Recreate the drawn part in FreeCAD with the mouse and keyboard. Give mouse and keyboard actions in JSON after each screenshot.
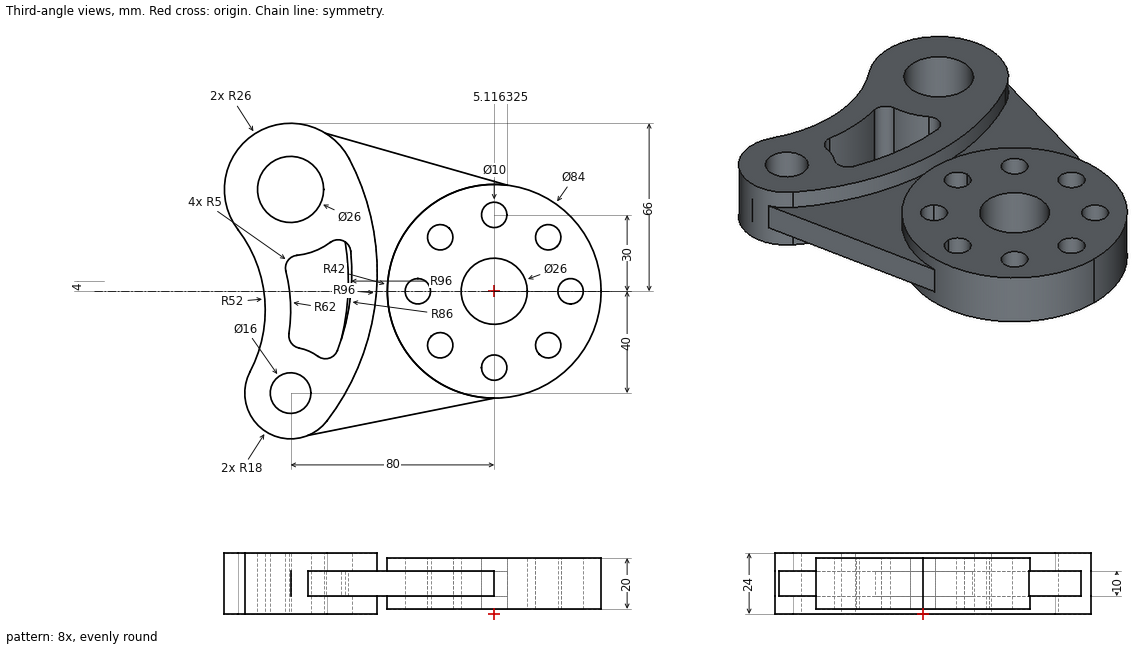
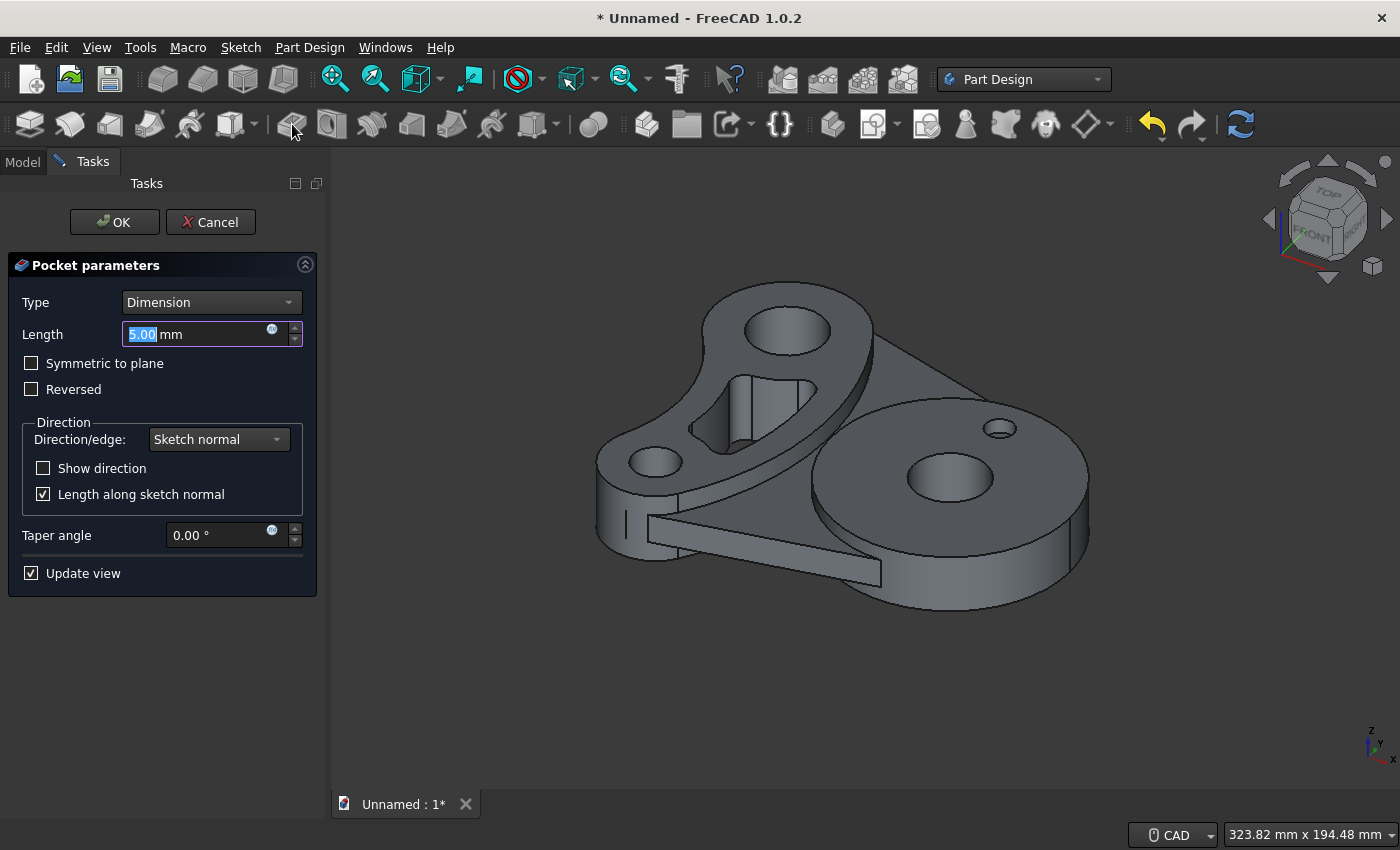
{"action": "left_click", "coordinate": [212, 302]}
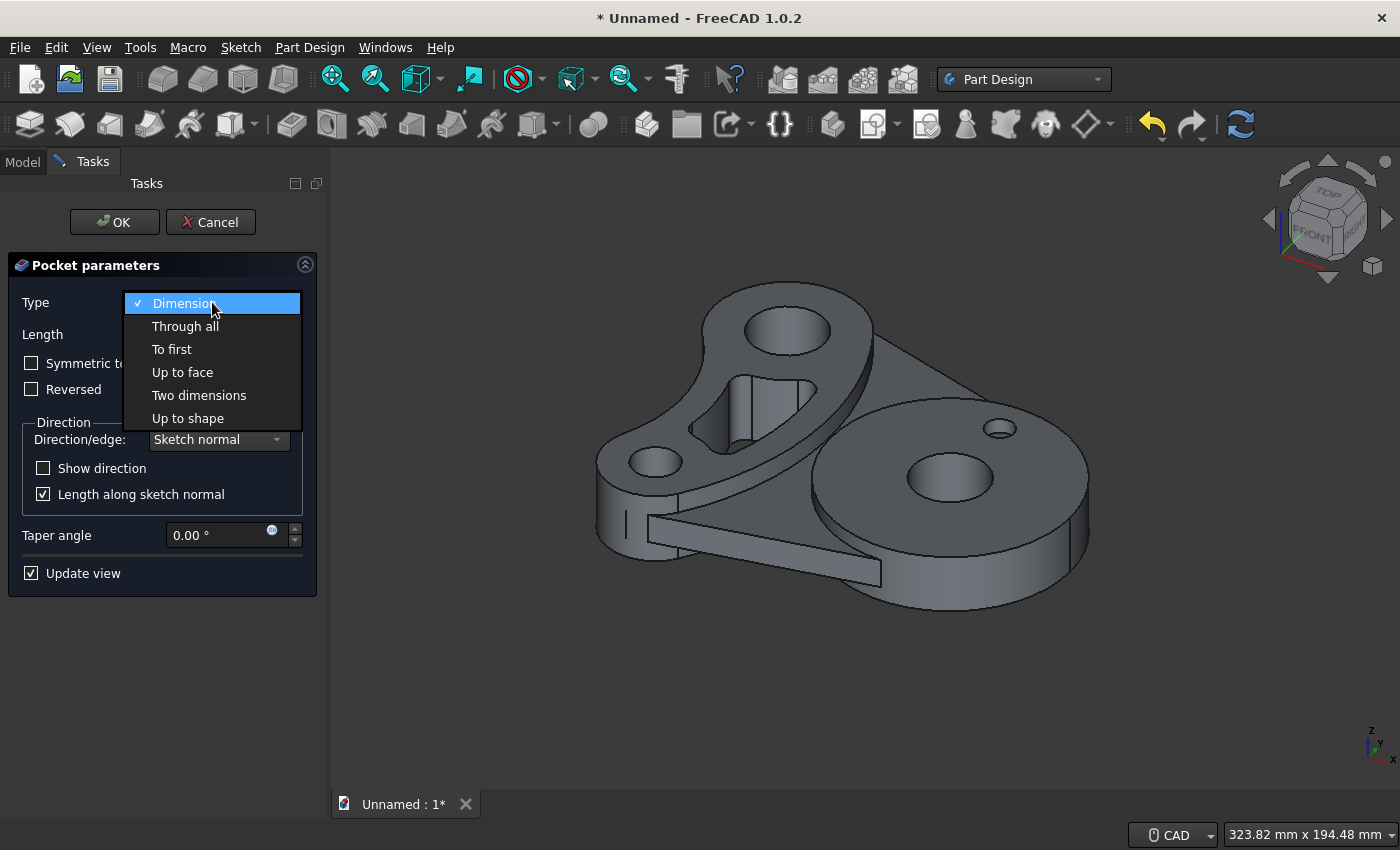
{"action": "left_click", "coordinate": [212, 326]}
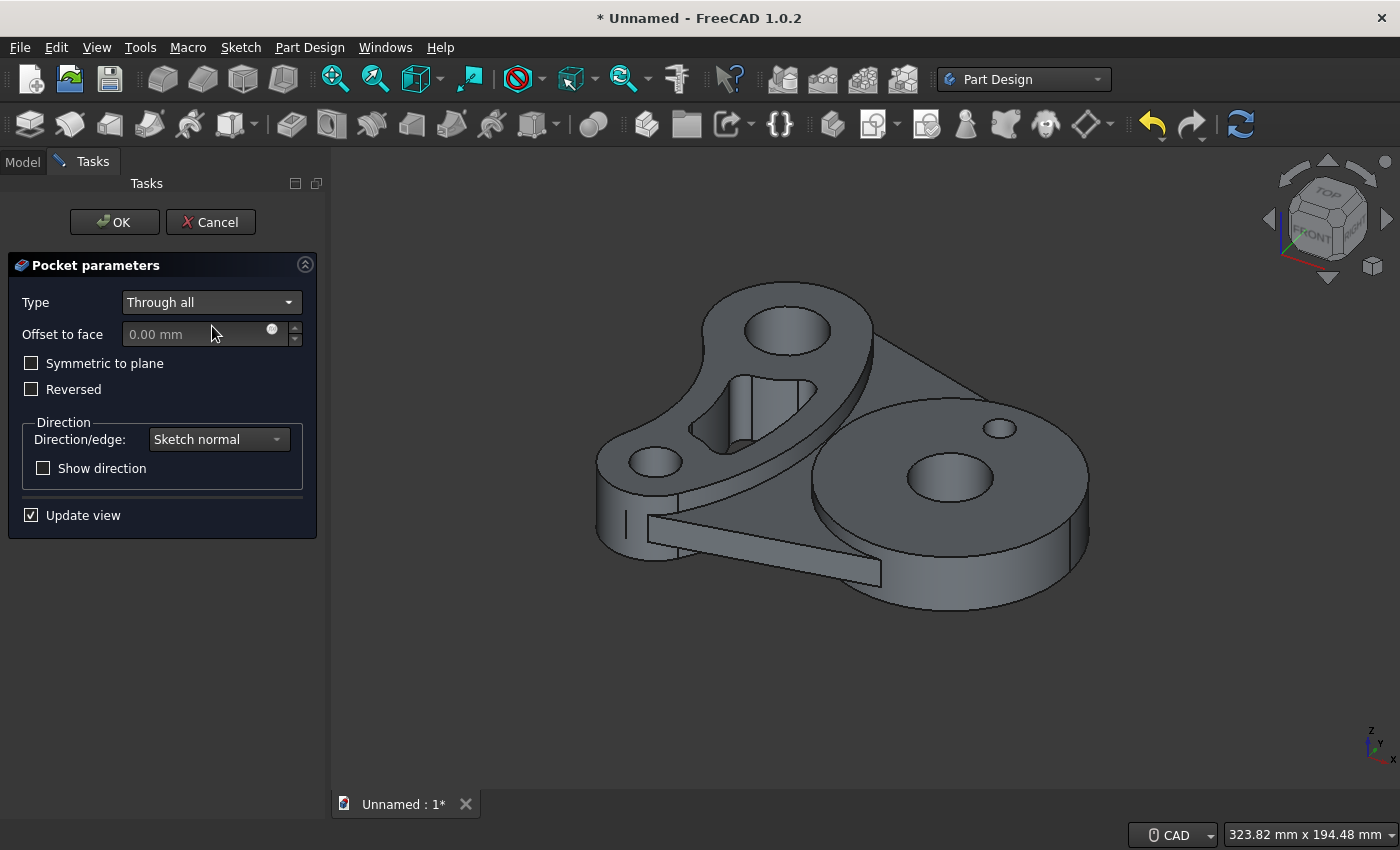
{"action": "left_click", "coordinate": [115, 222]}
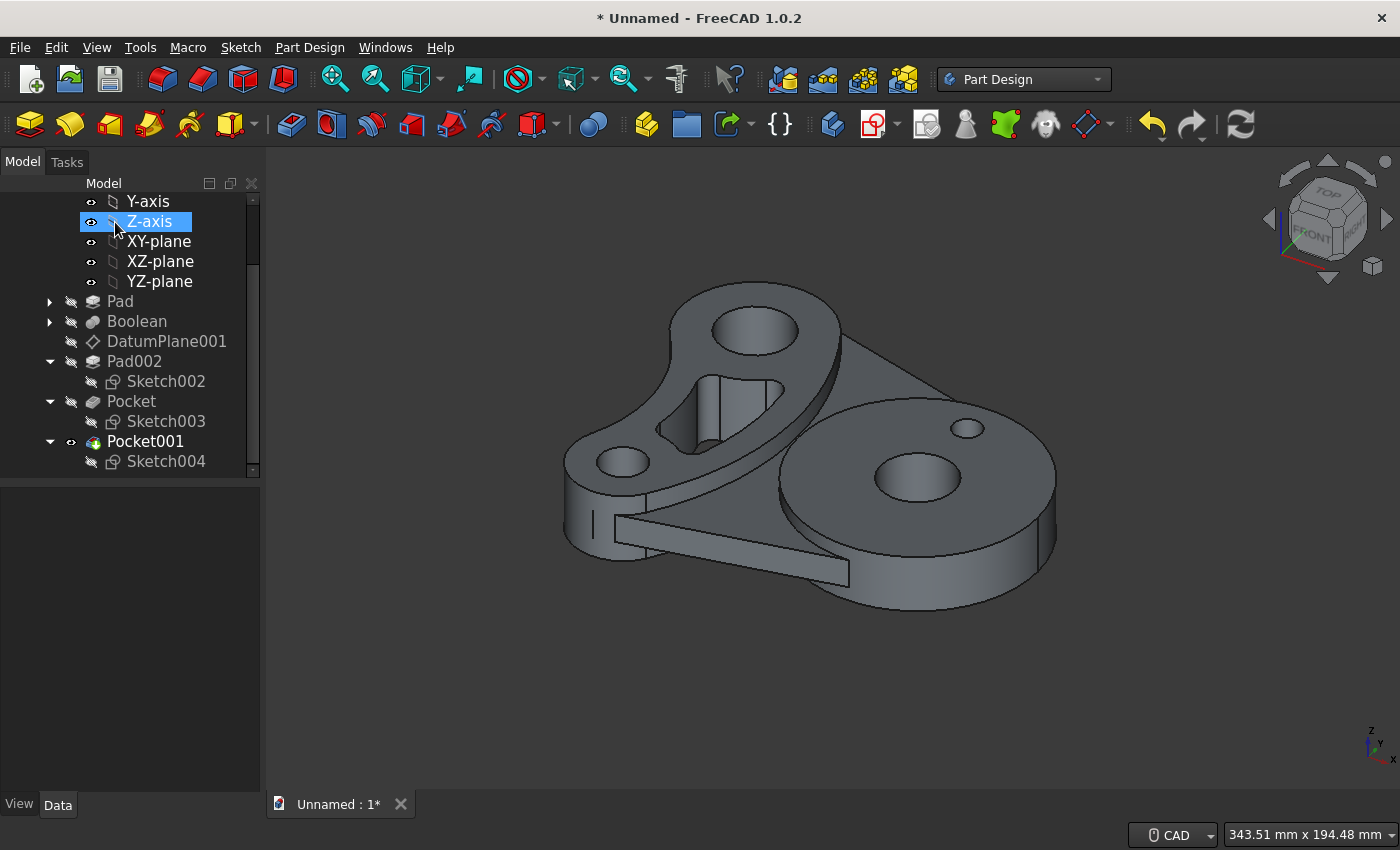
{"action": "left_click", "coordinate": [116, 442]}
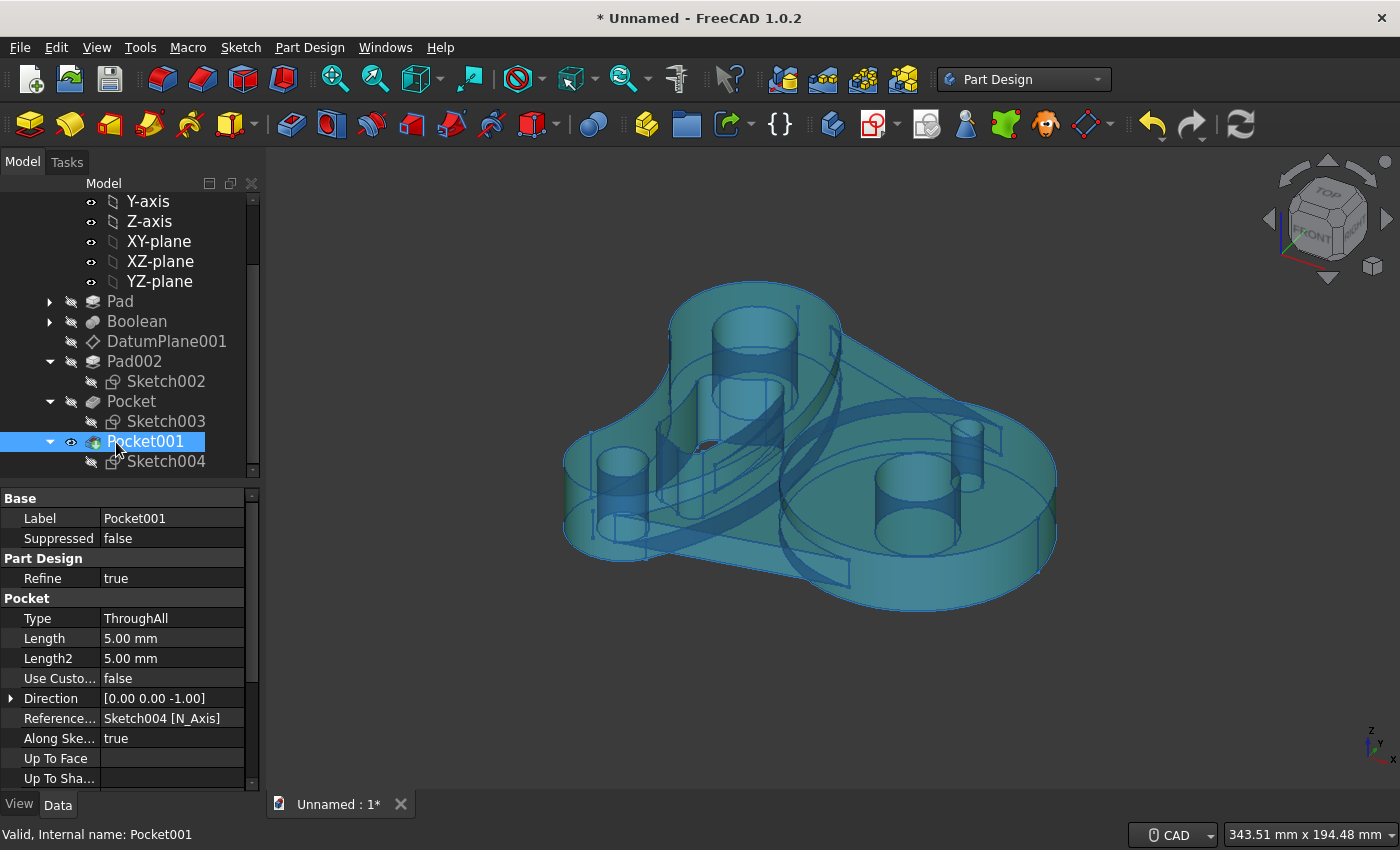
{"action": "left_click", "coordinate": [864, 80]}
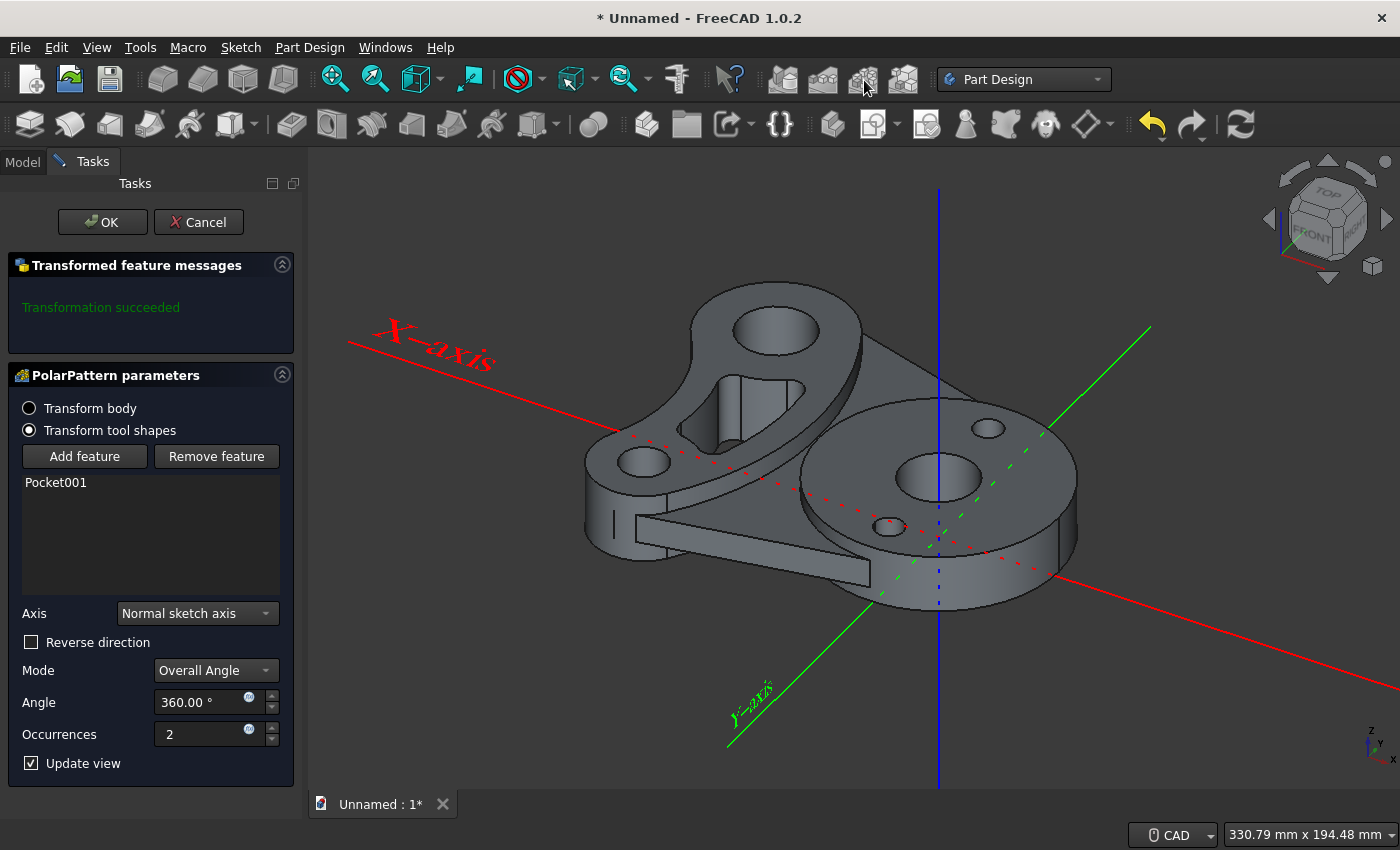
{"action": "left_click", "coordinate": [198, 614]}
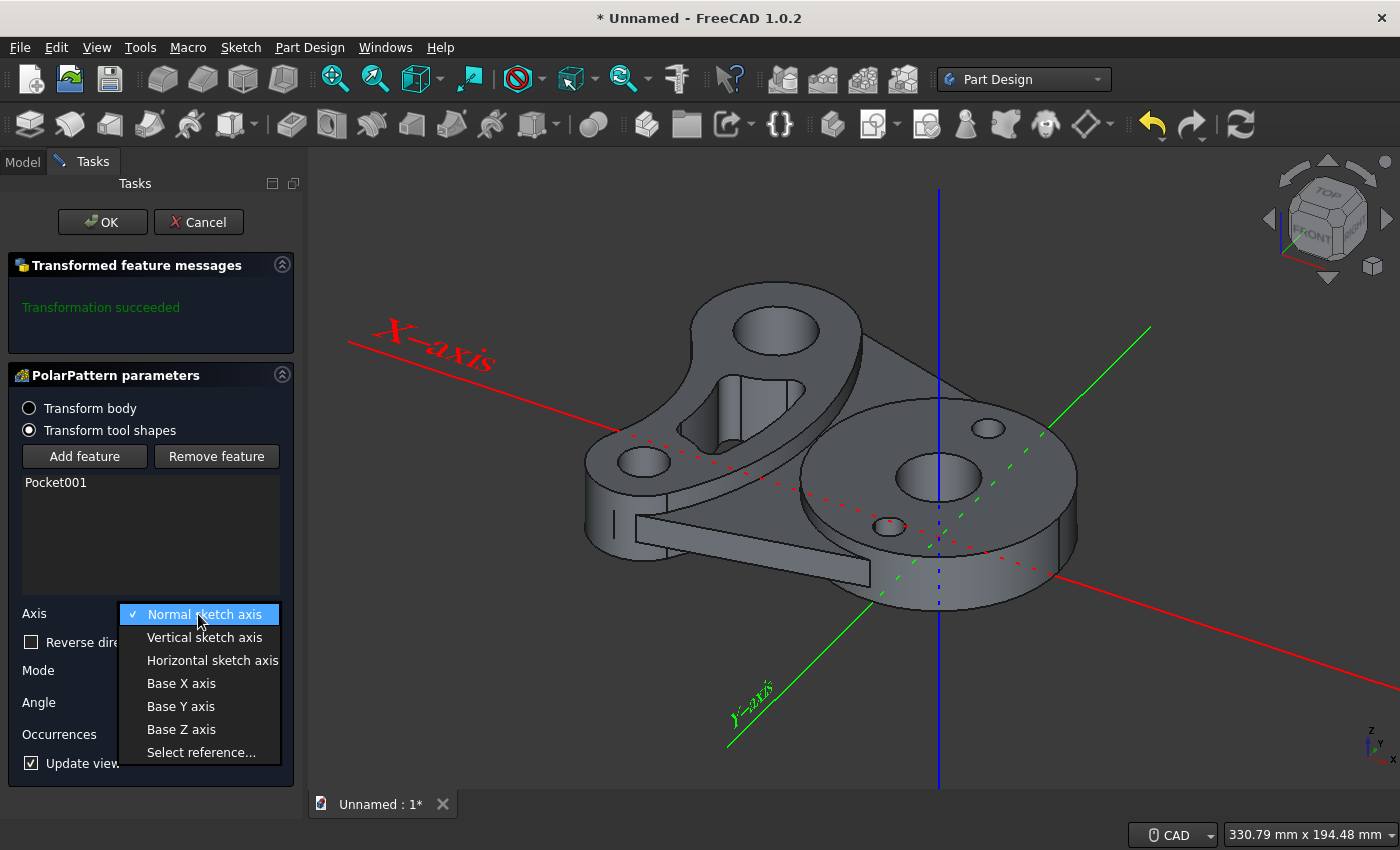
{"action": "left_click", "coordinate": [198, 730]}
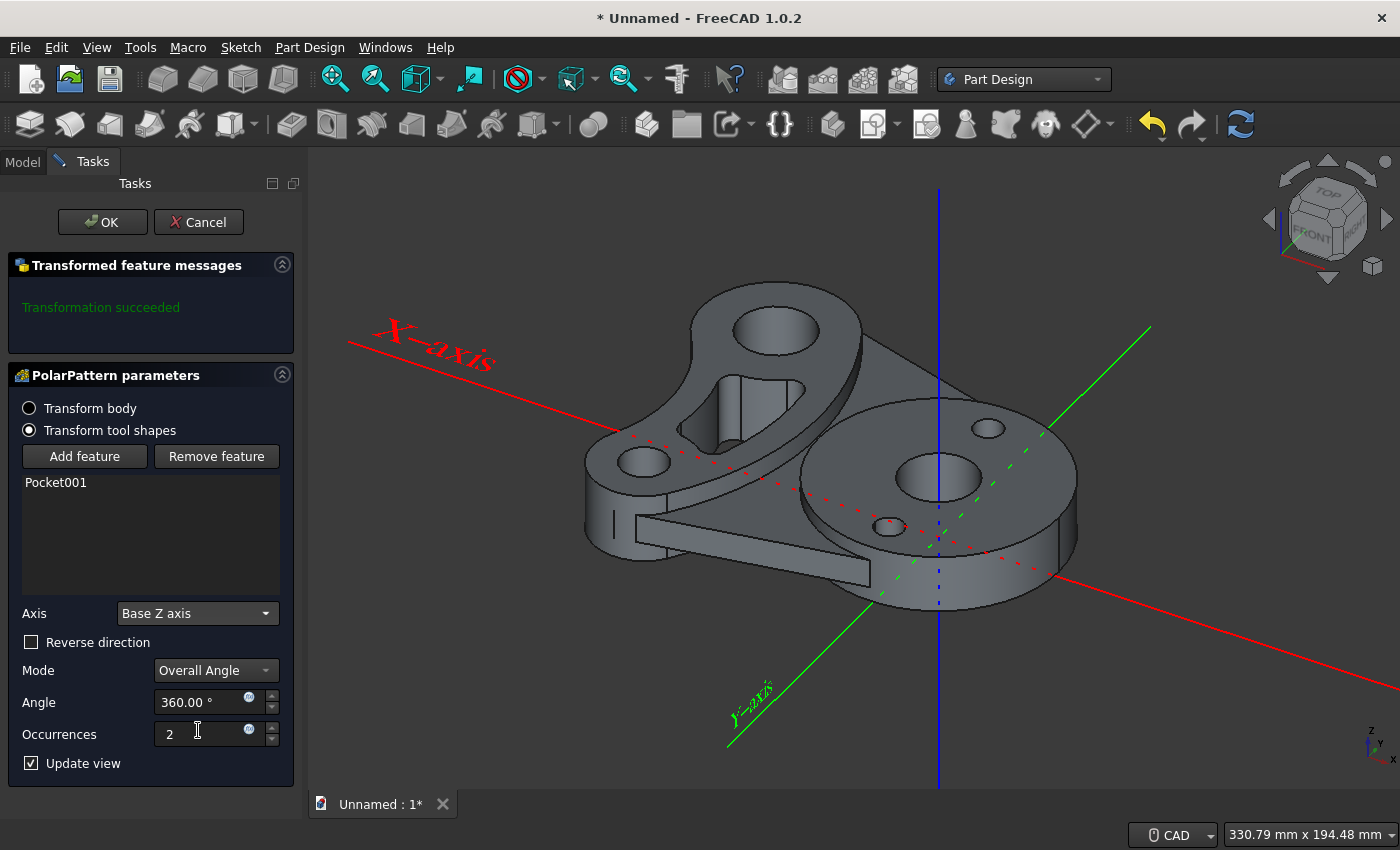
{"action": "triple_click", "coordinate": [209, 734]}